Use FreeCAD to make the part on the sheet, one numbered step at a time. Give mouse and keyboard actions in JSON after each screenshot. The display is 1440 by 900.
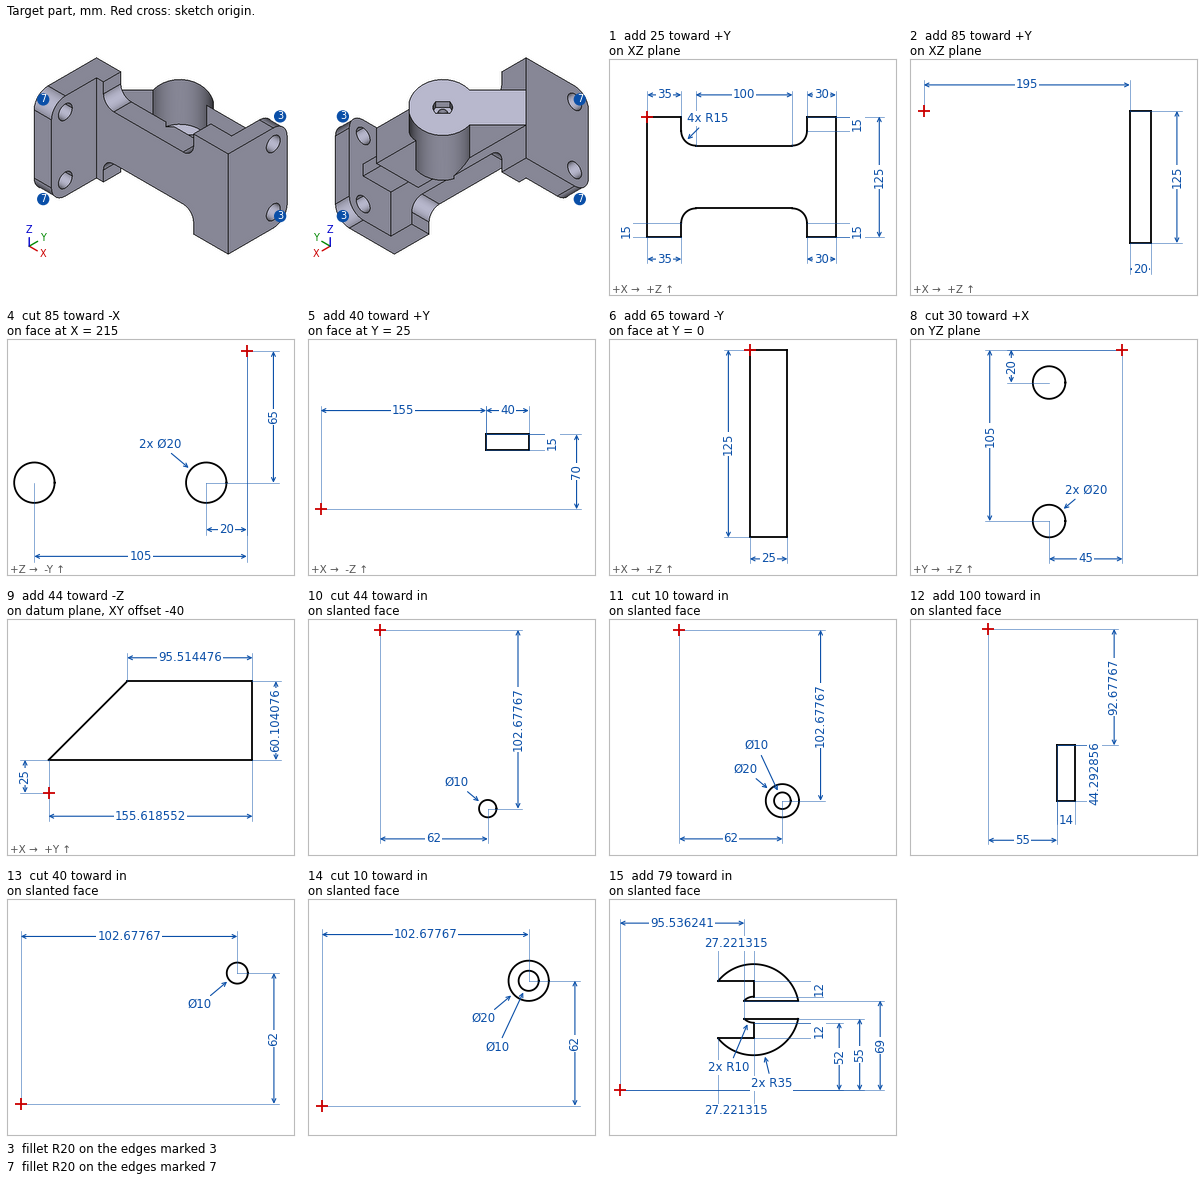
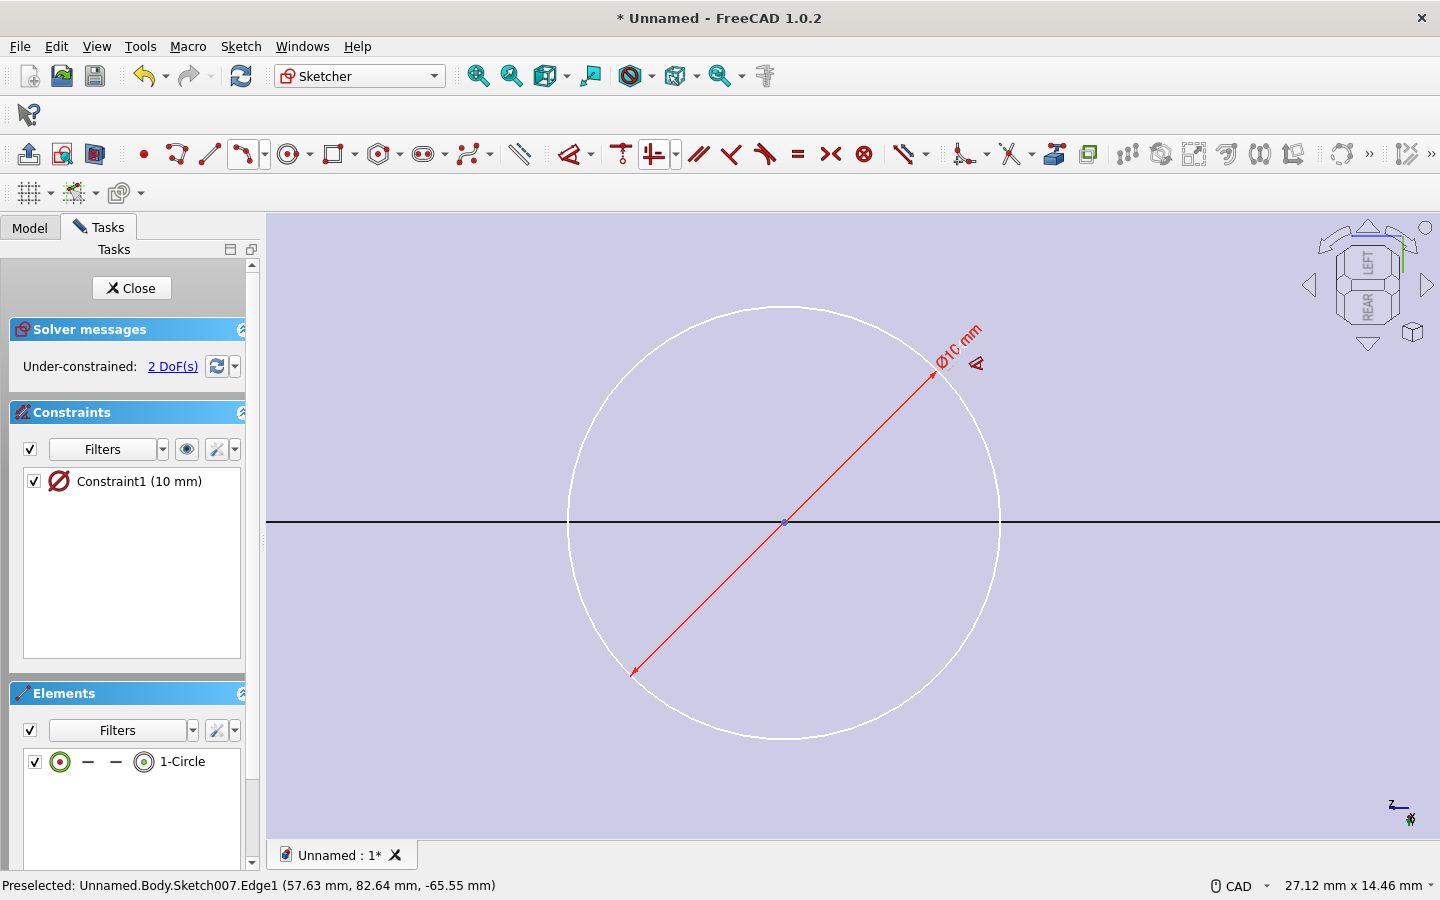
{"action": "left_click", "coordinate": [784, 523]}
{"action": "left_click", "coordinate": [539, 557]}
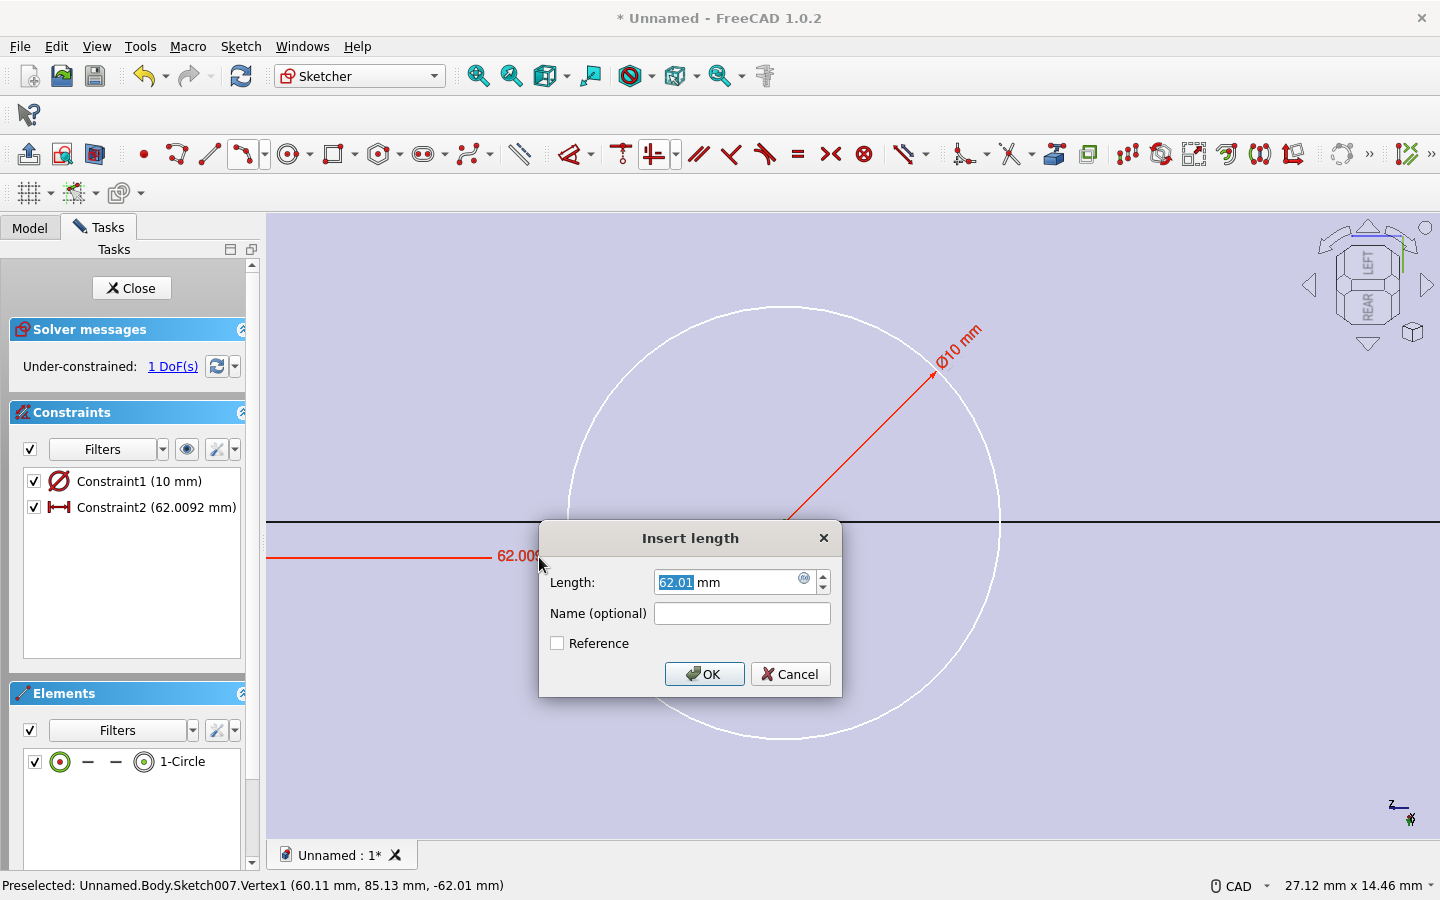
{"action": "type", "text": "62"}
{"action": "key", "text": "Return"}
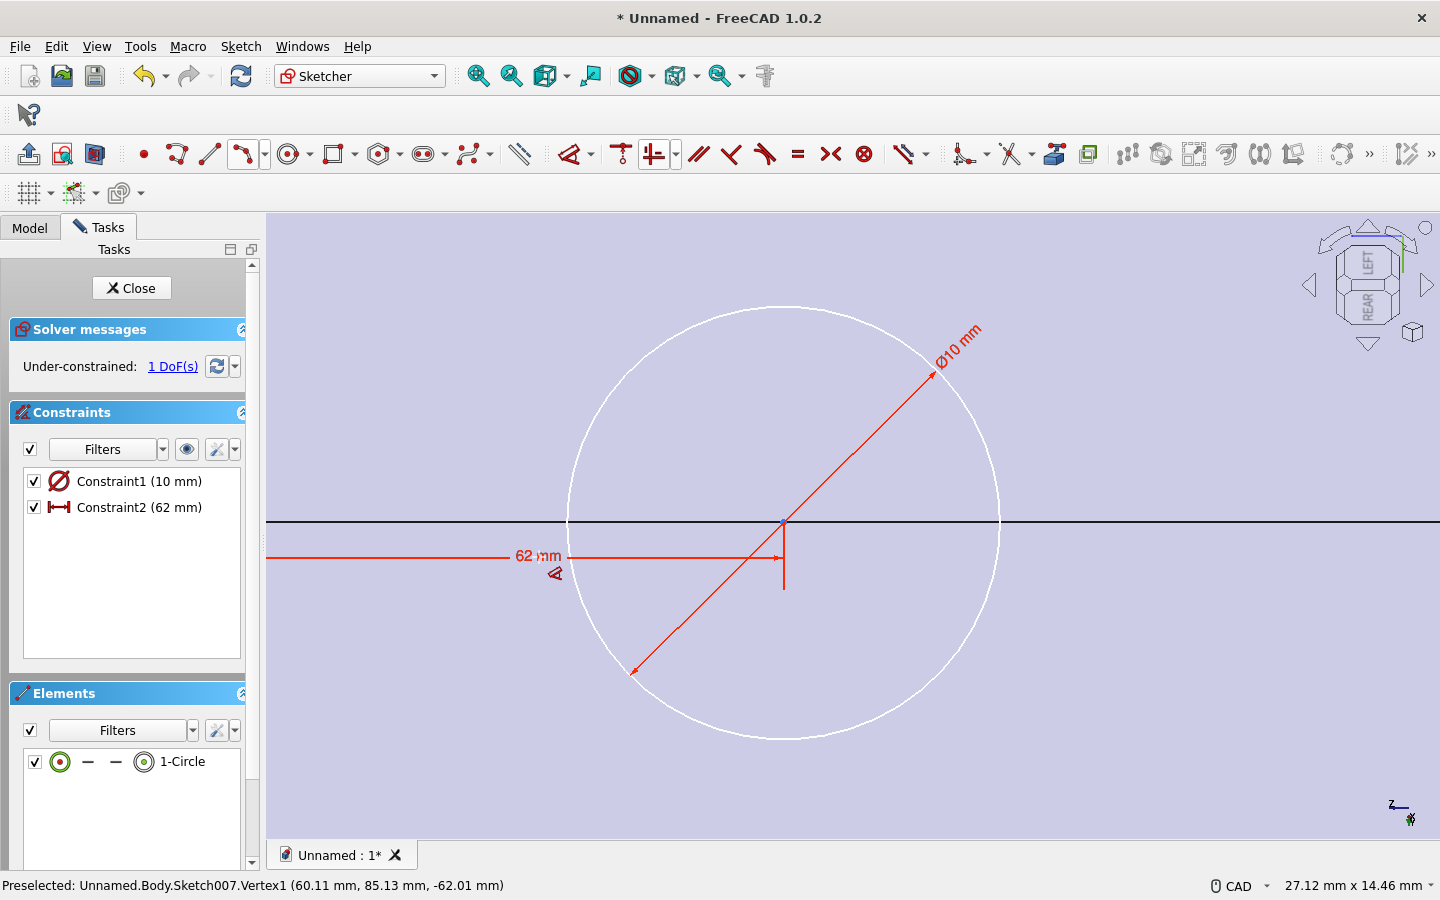
{"action": "left_click", "coordinate": [784, 523]}
{"action": "left_click", "coordinate": [818, 382]}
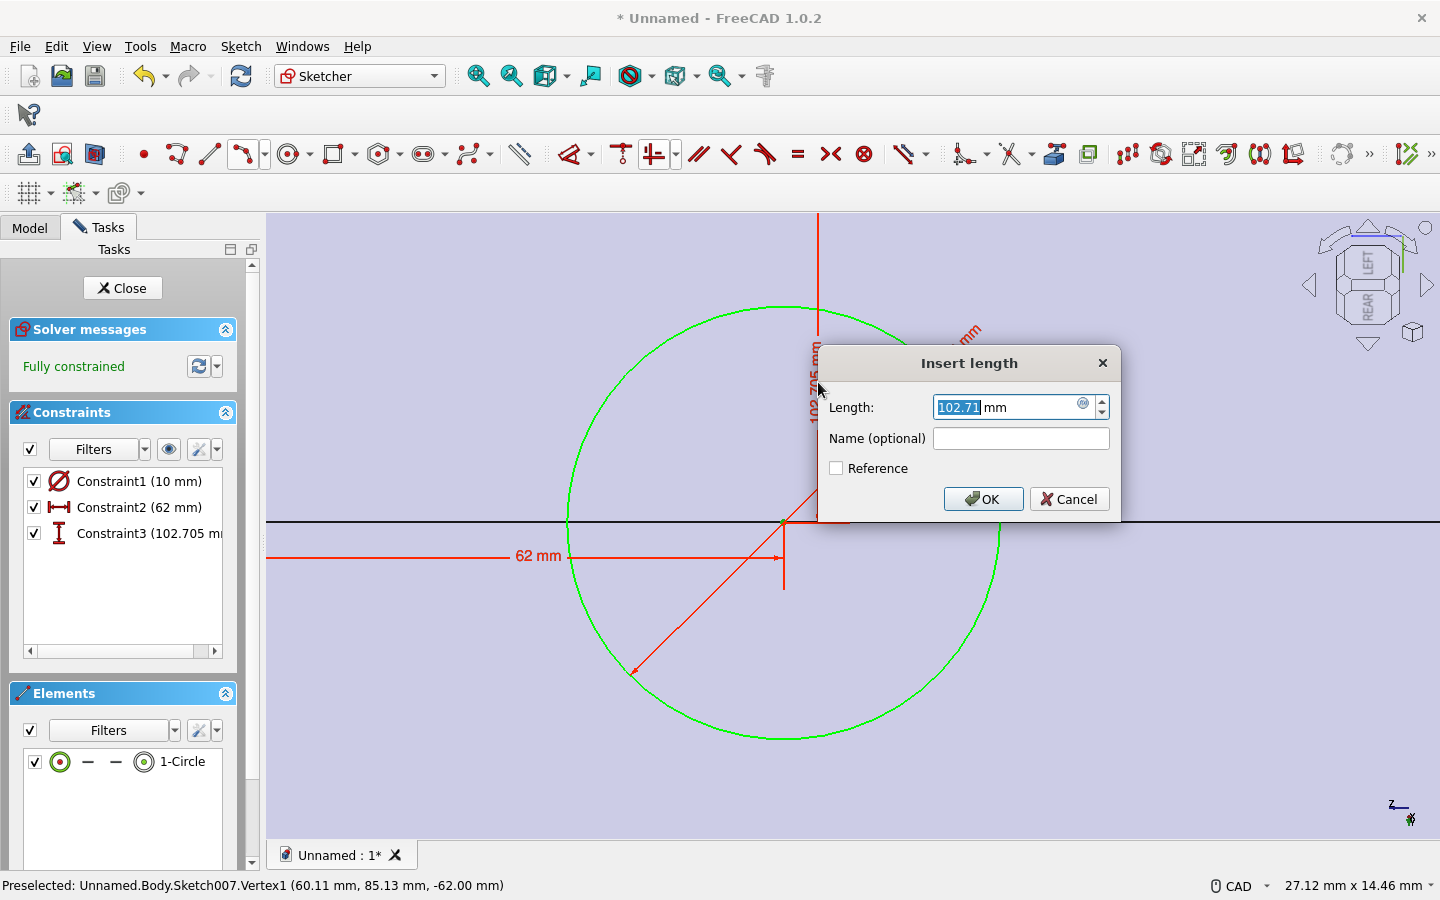
{"action": "type", "text": "102.67767"}
{"action": "key", "text": "Return"}
{"action": "key", "text": "Escape"}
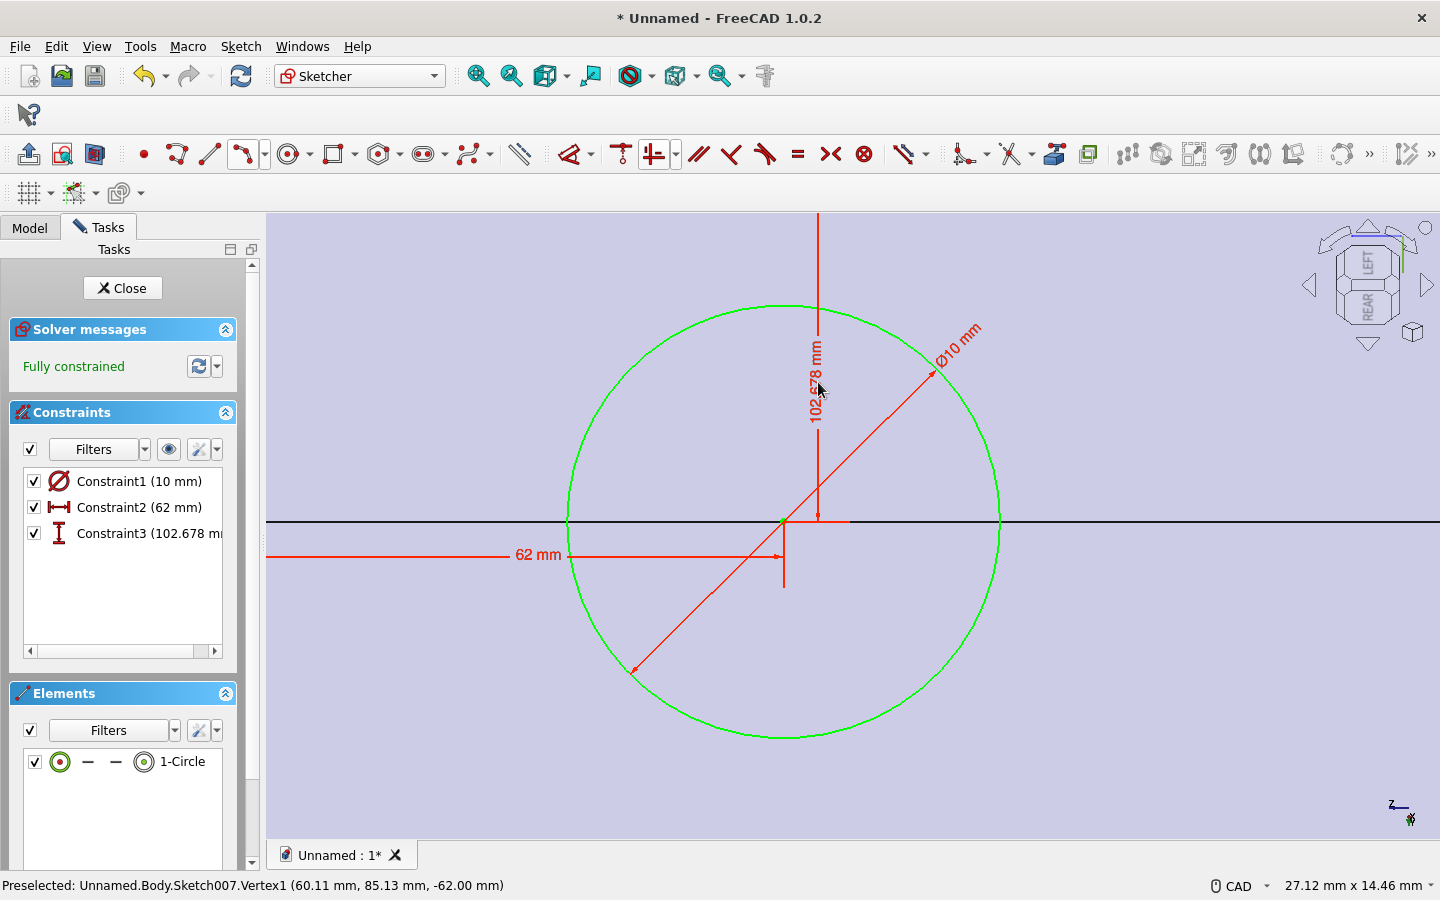
{"action": "left_click", "coordinate": [123, 288]}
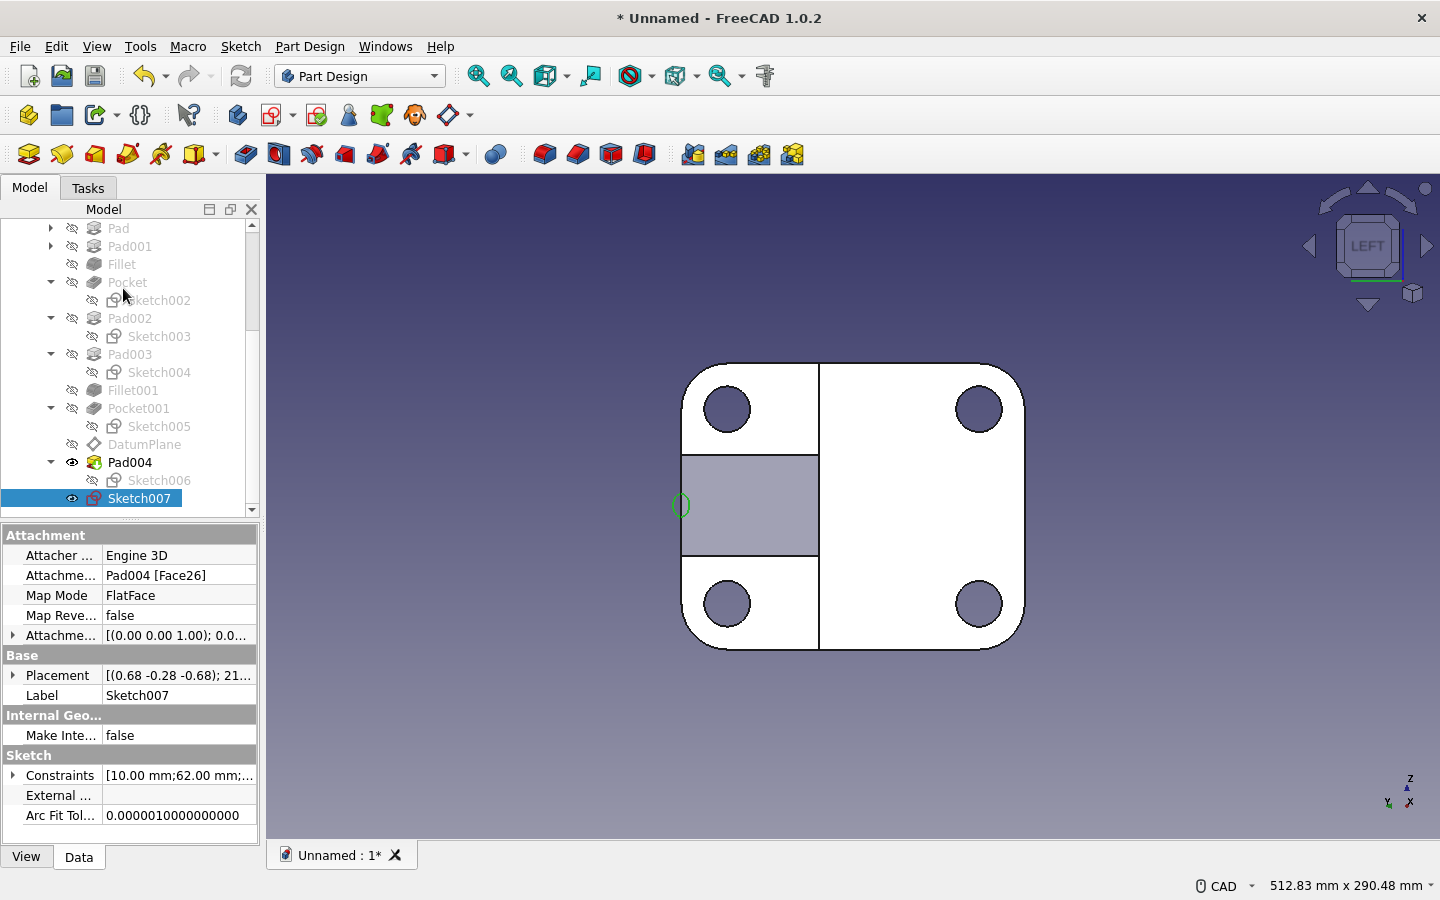
{"action": "left_click", "coordinate": [246, 154]}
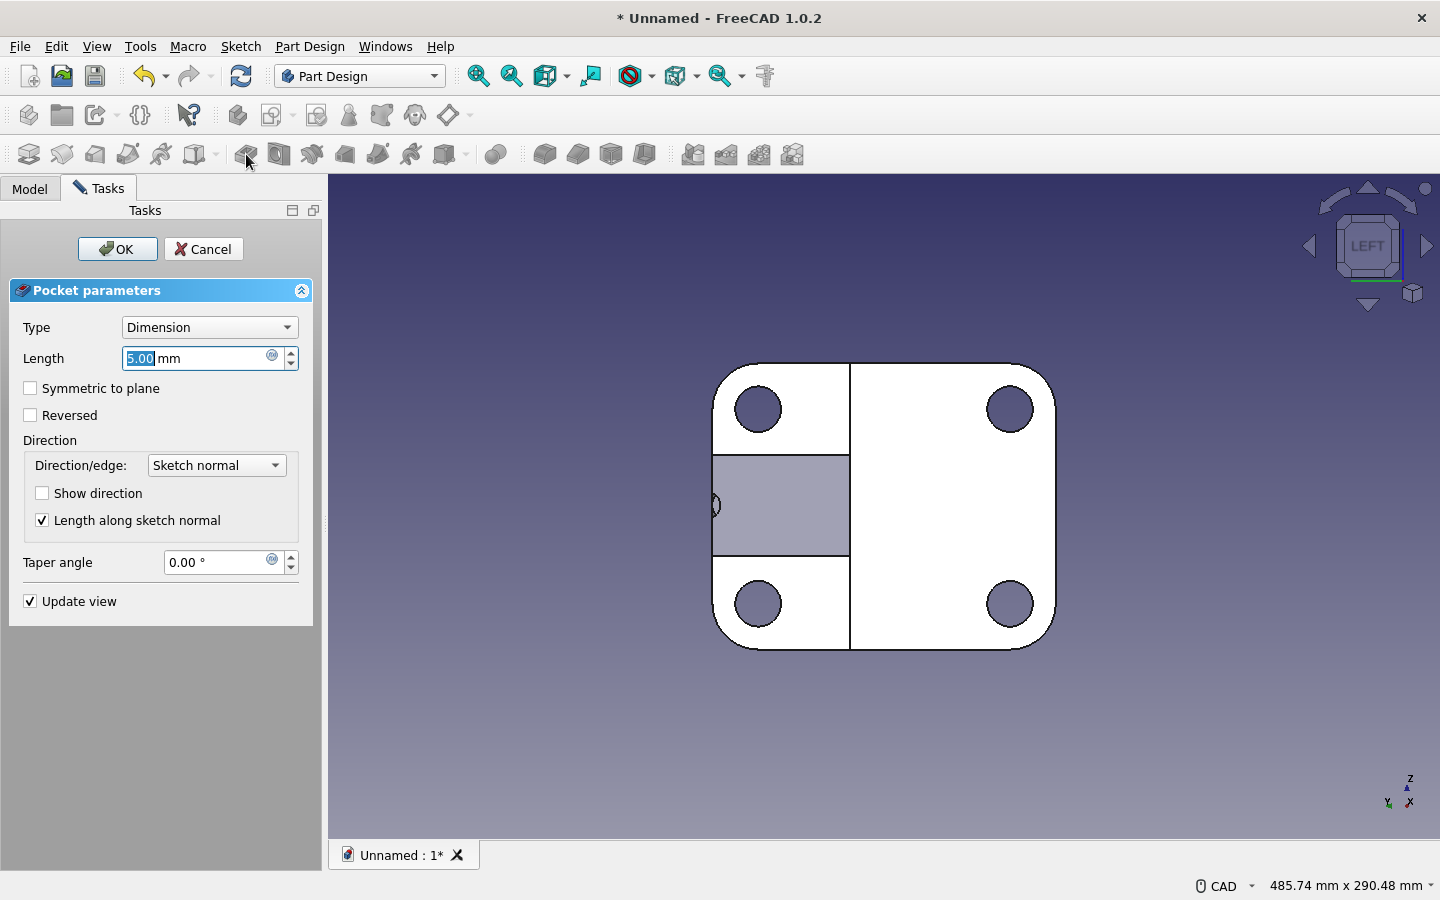
{"action": "type", "text": "44"}
{"action": "key", "text": "Tab"}